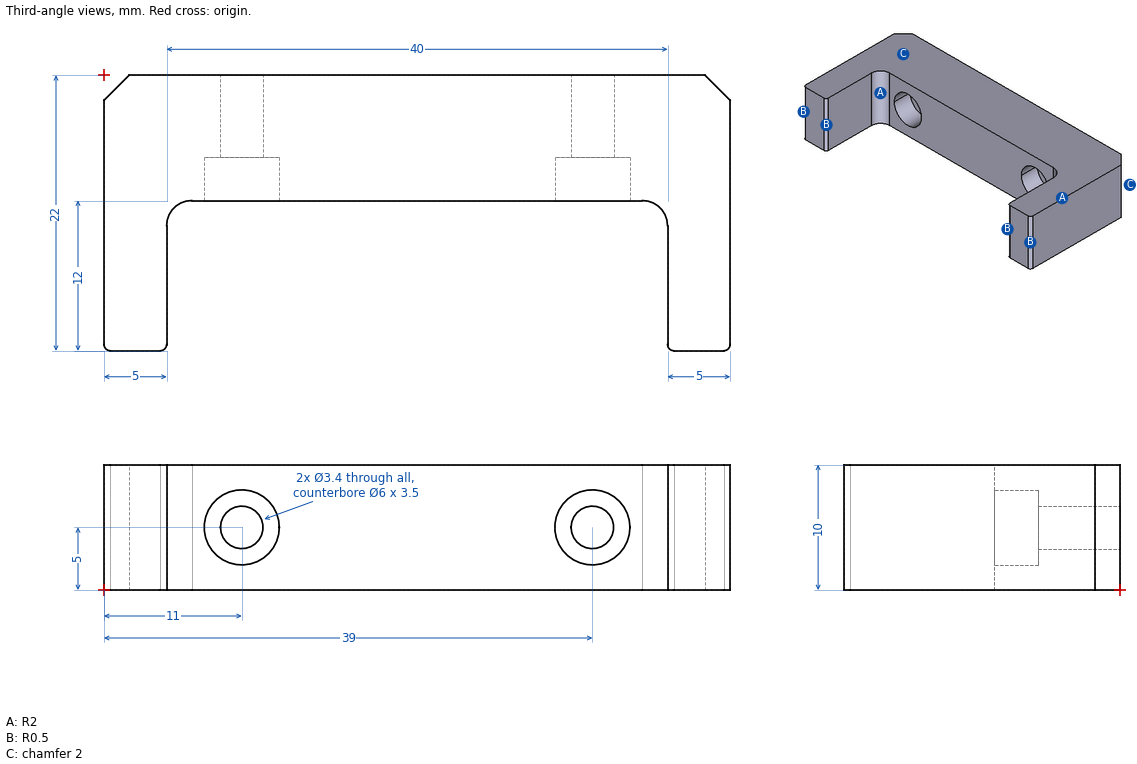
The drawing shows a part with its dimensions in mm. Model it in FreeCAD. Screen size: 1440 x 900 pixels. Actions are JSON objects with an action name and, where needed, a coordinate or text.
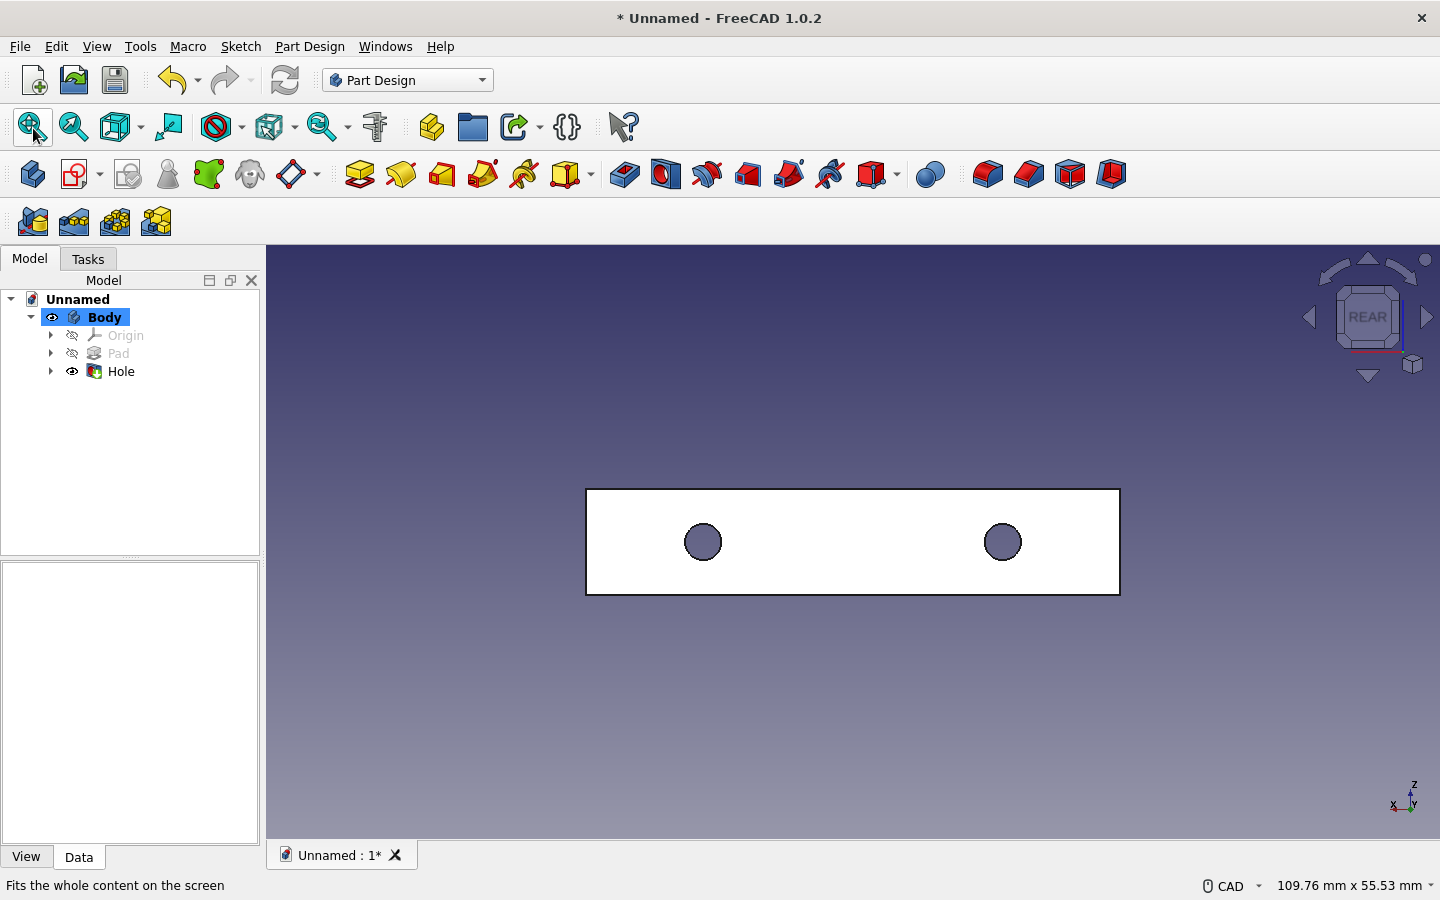
{"action": "key", "text": "6"}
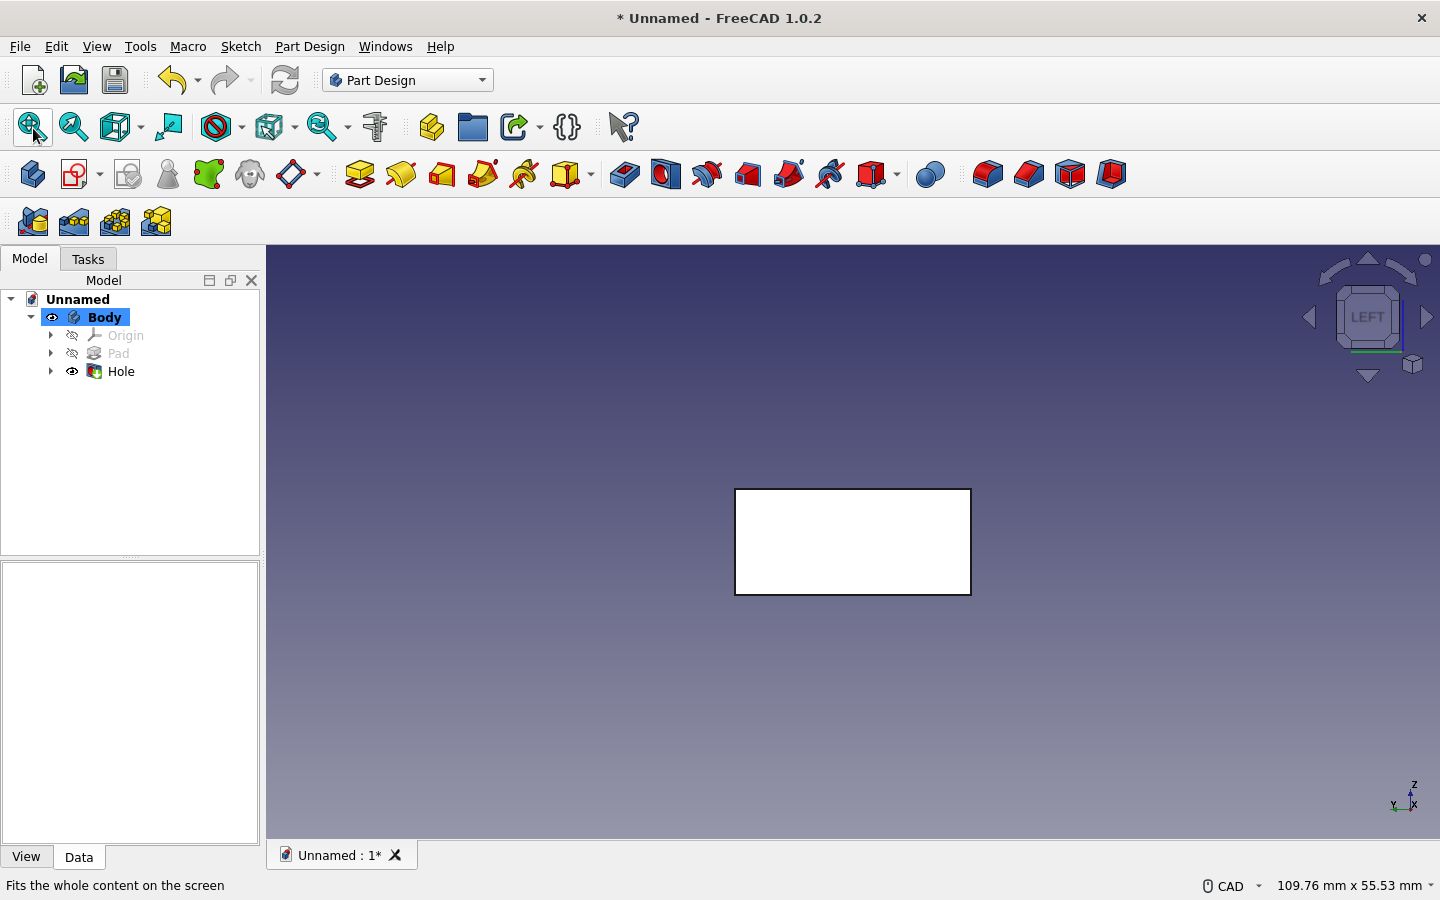
{"action": "left_click", "coordinate": [33, 128]}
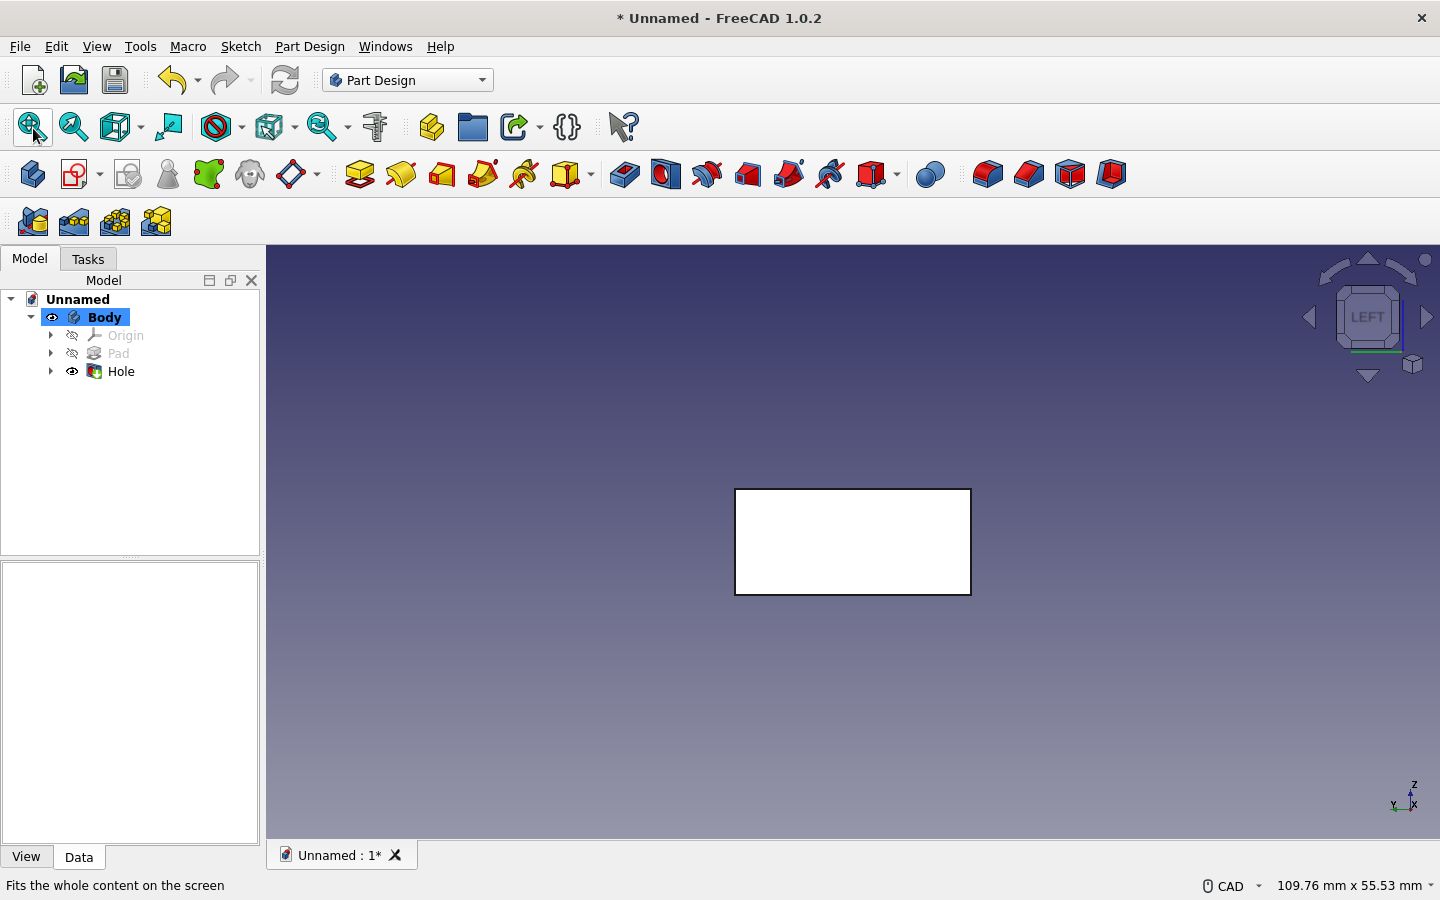
{"action": "key", "text": "v 3"}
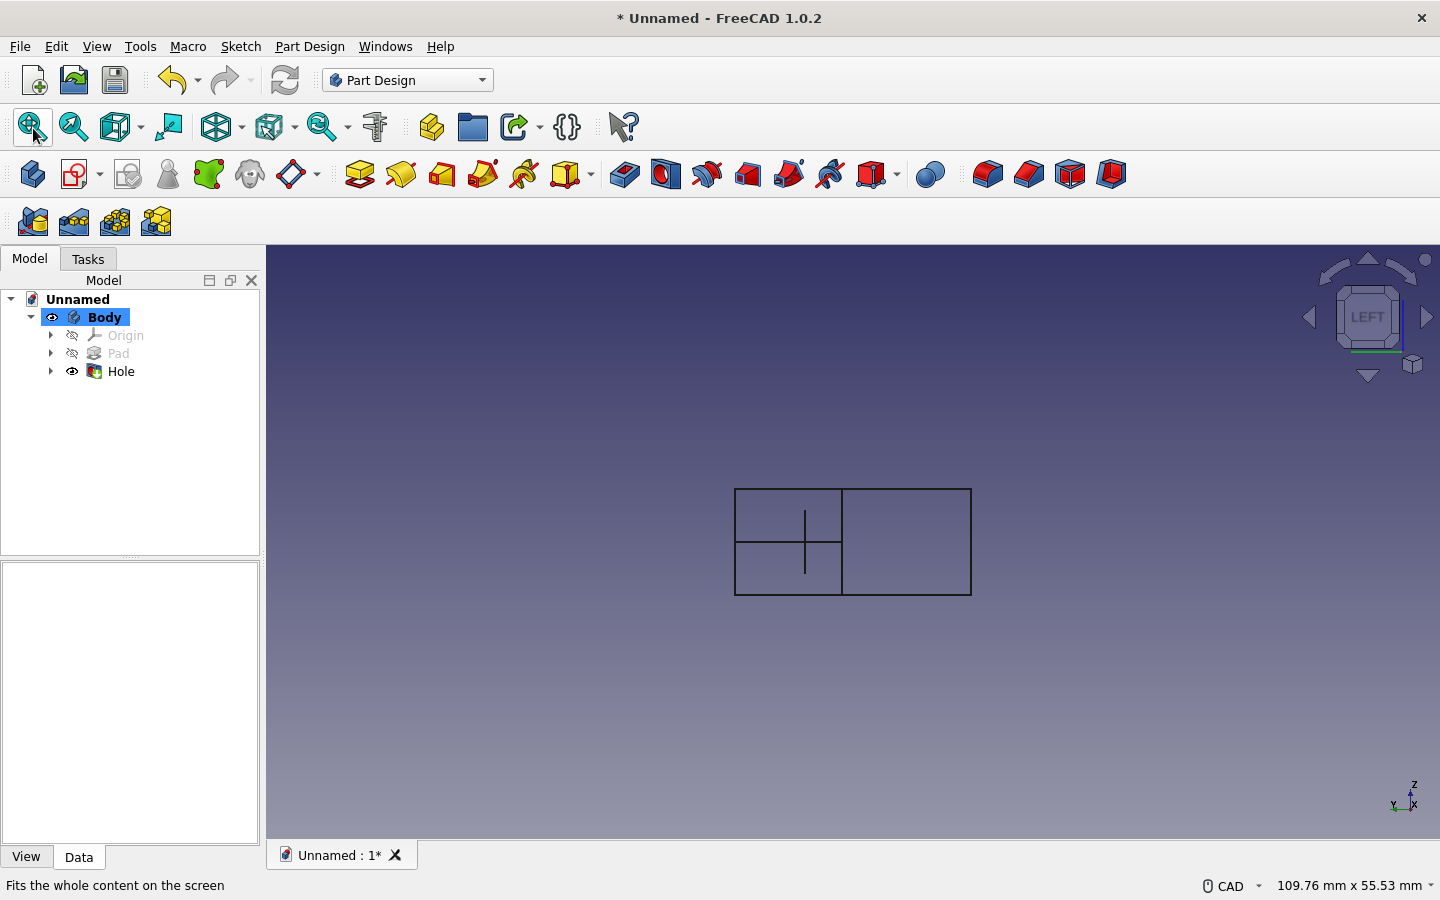
{"action": "key", "text": "0"}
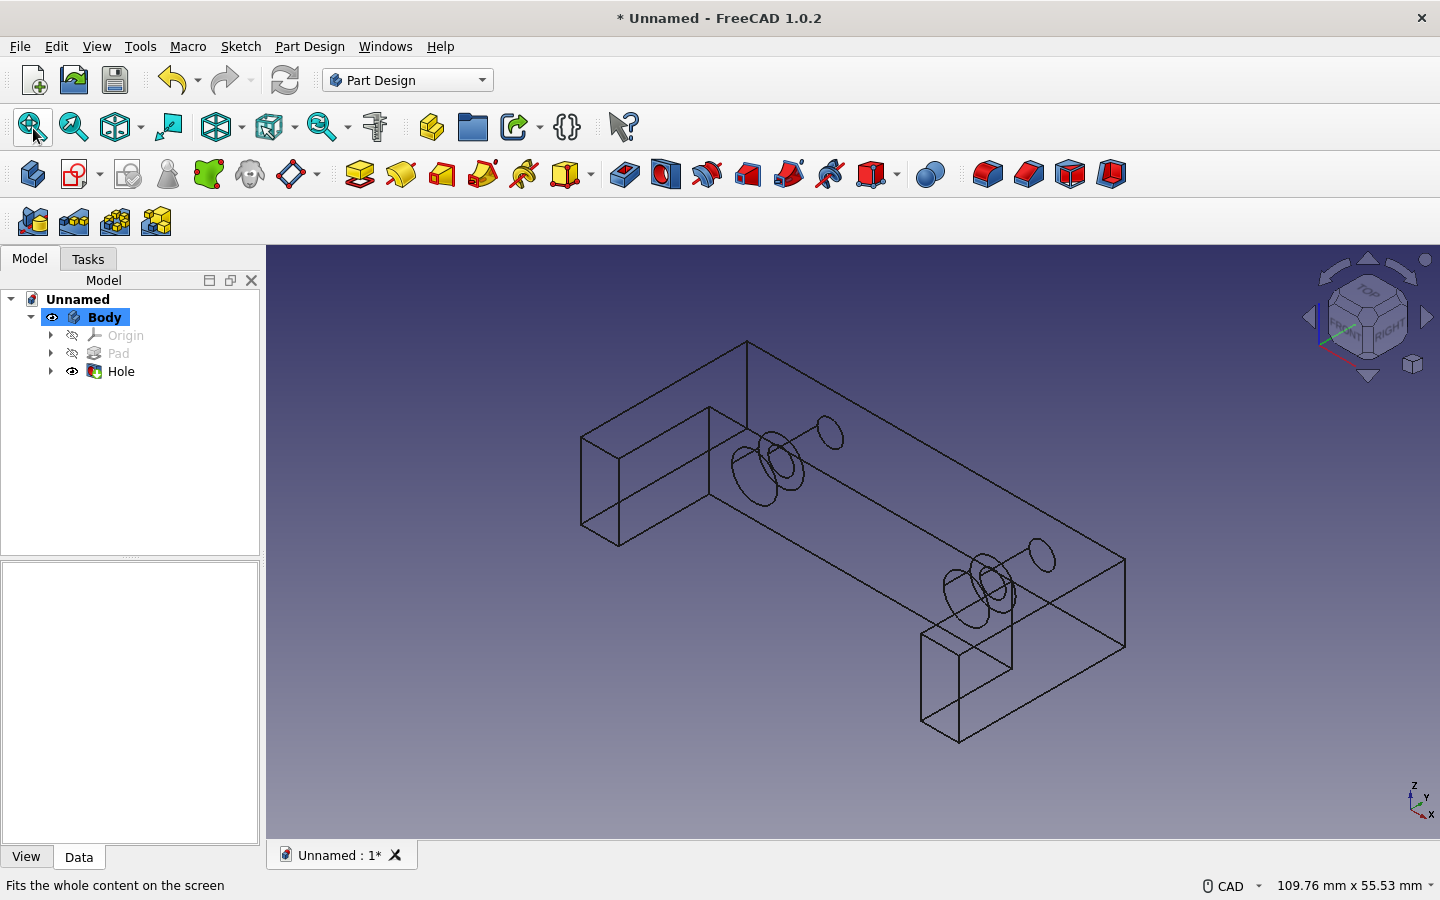
{"action": "left_click", "coordinate": [1012, 633]}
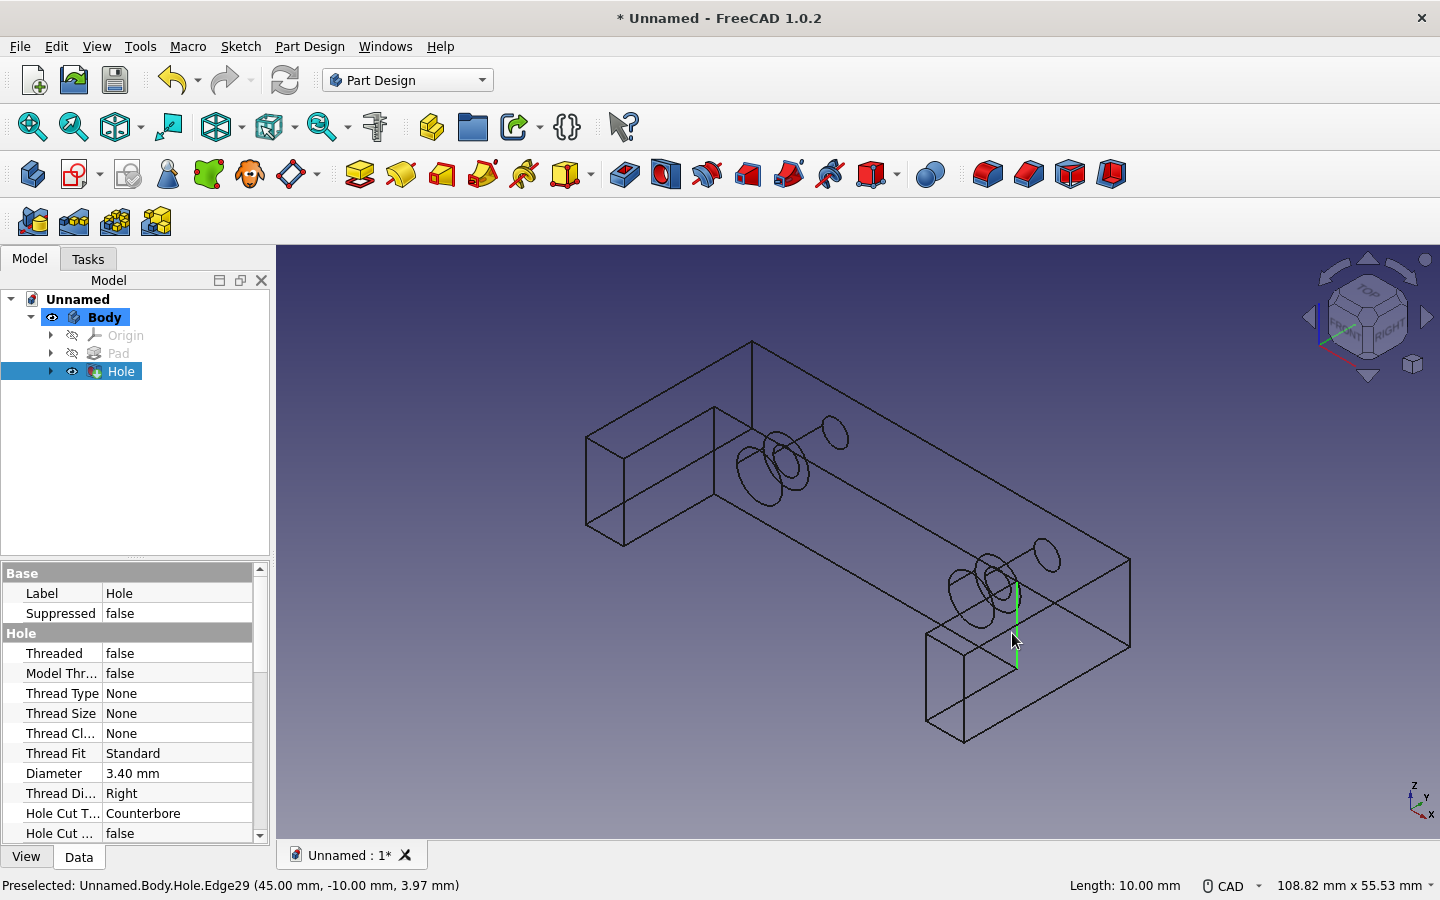
{"action": "left_click", "coordinate": [714, 449], "text": "ctrl"}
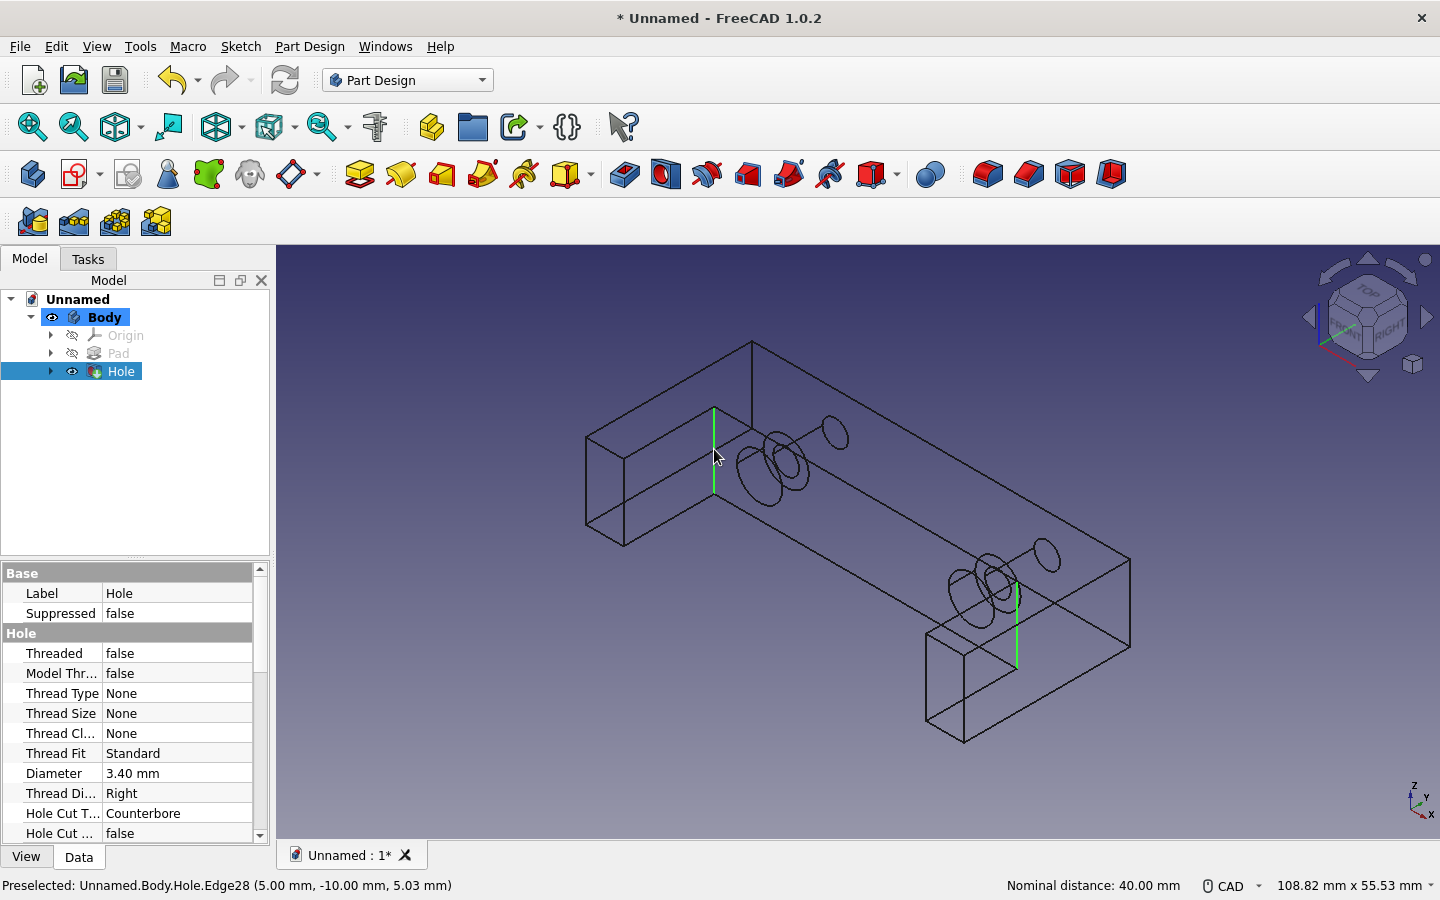
{"action": "key", "text": "v 1"}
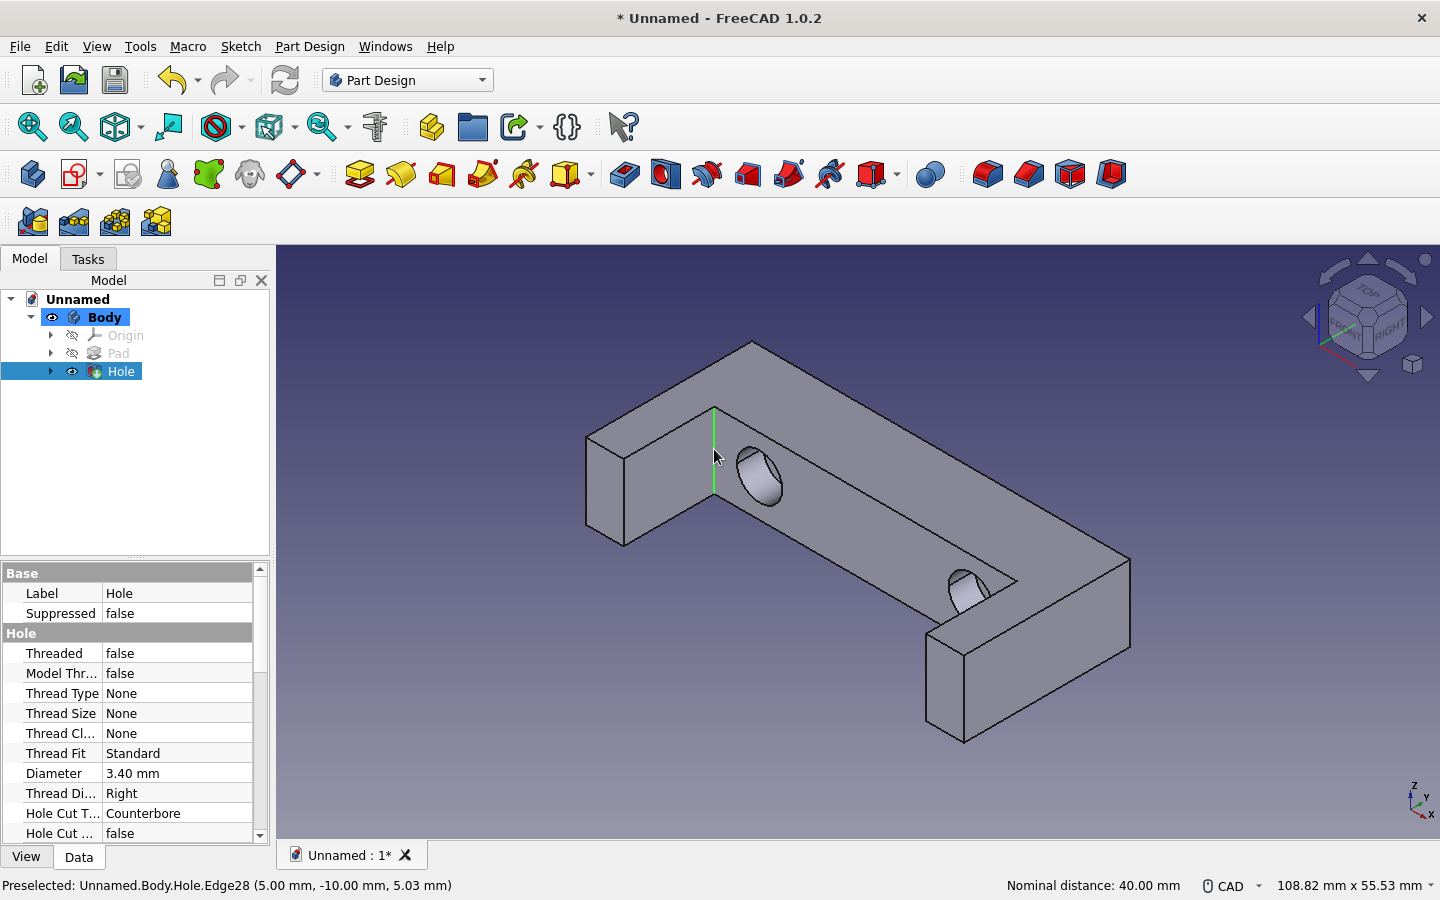
{"action": "left_click", "coordinate": [988, 174]}